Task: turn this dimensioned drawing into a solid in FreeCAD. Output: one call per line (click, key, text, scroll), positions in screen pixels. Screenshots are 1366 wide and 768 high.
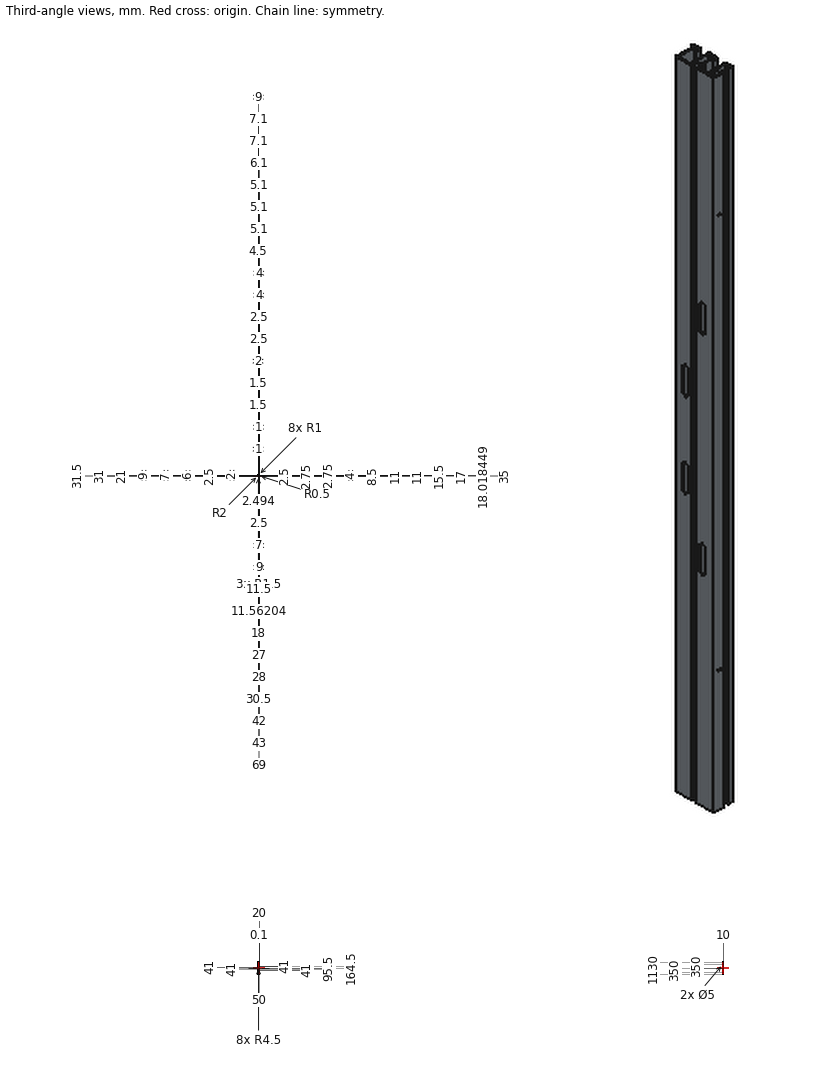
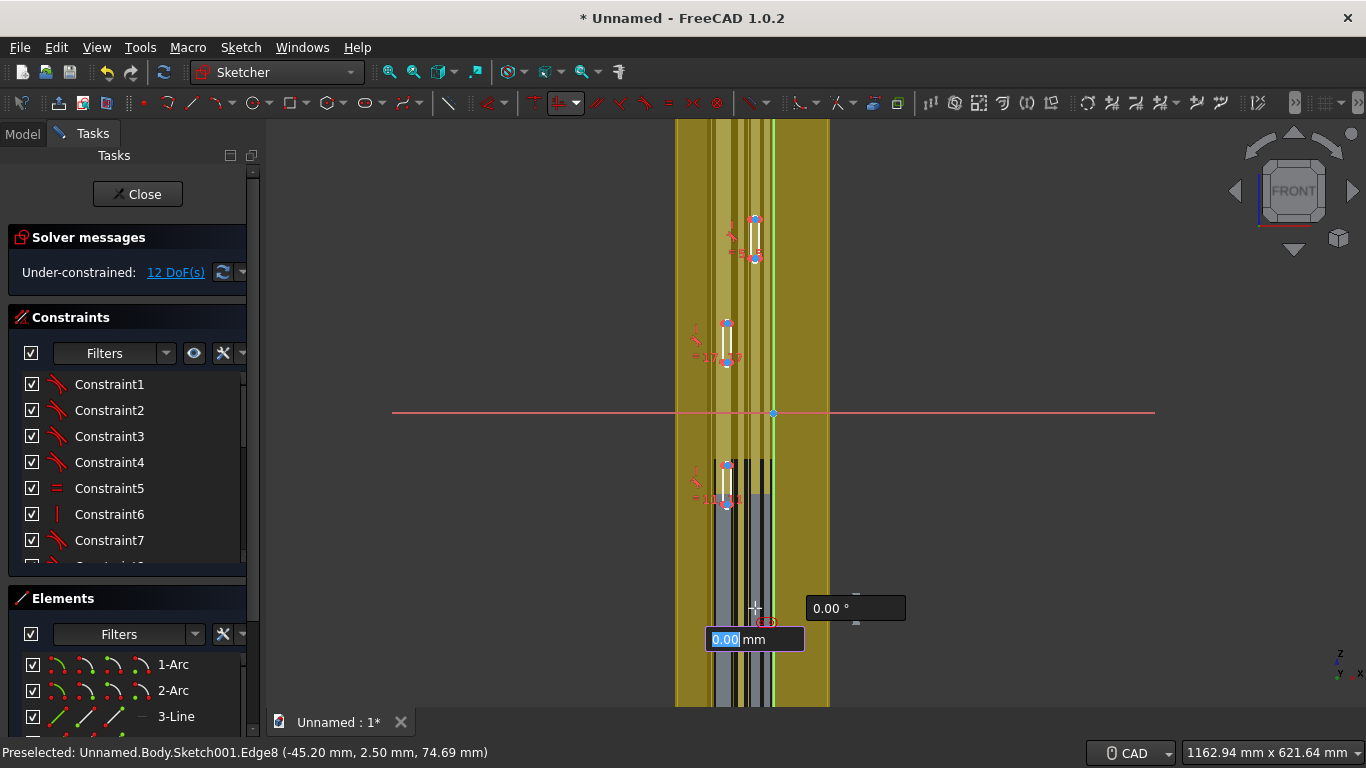
click(755, 569)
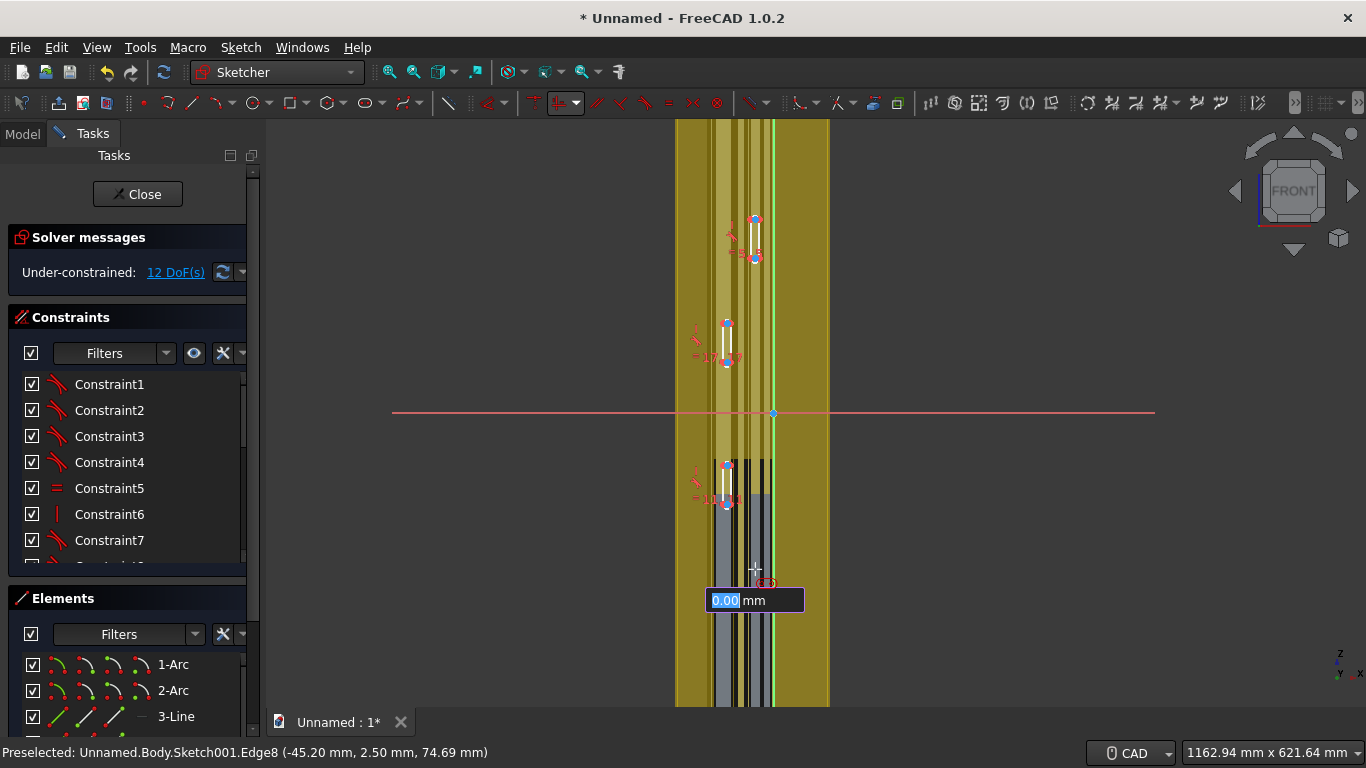
scroll(759, 588, up, 7)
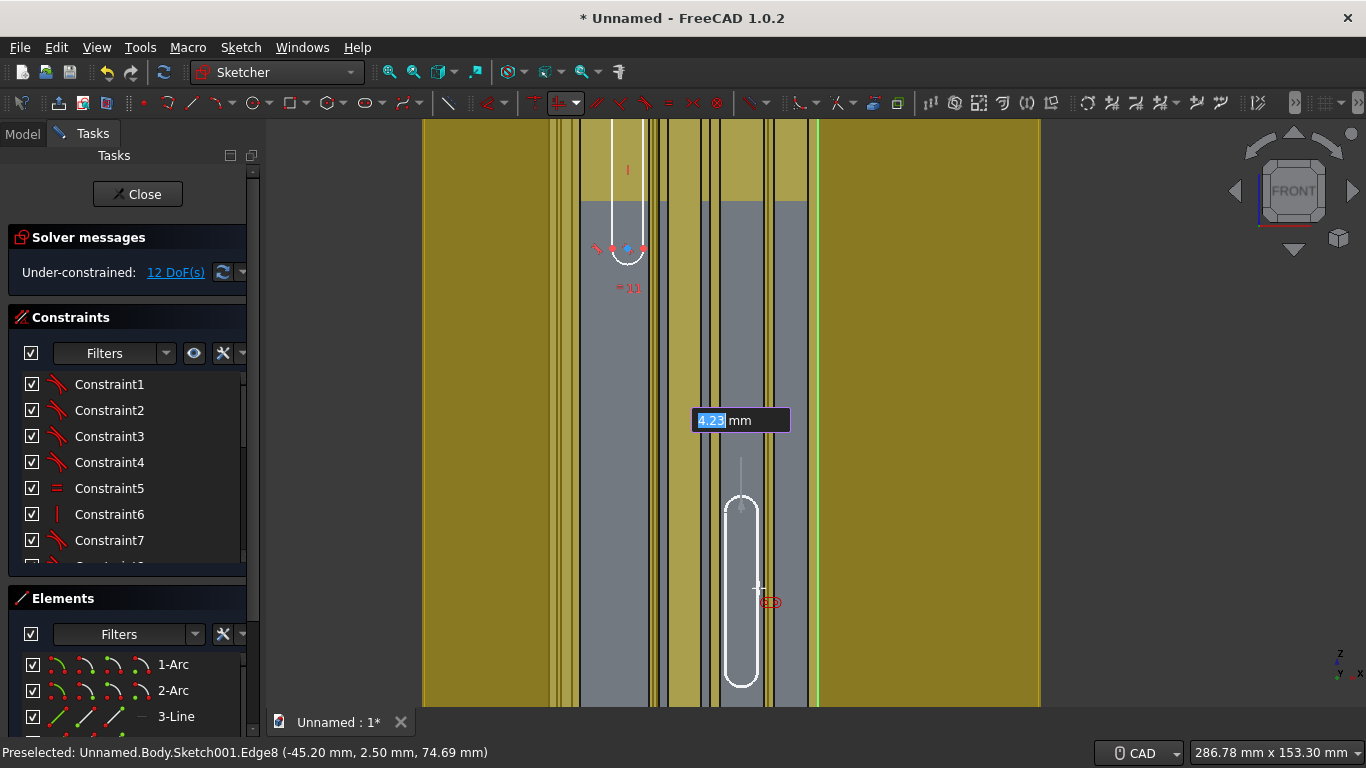
click(758, 587)
key(Escape)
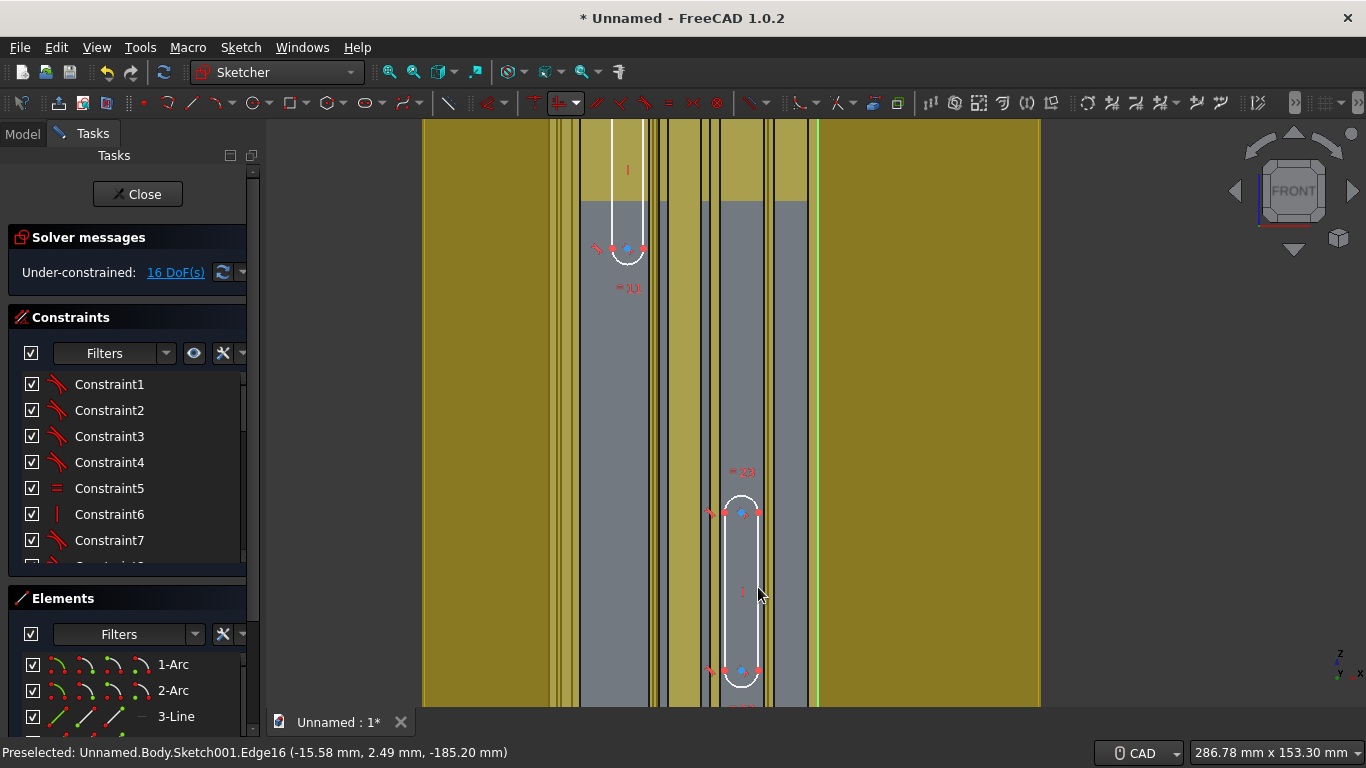
scroll(759, 588, down, 7)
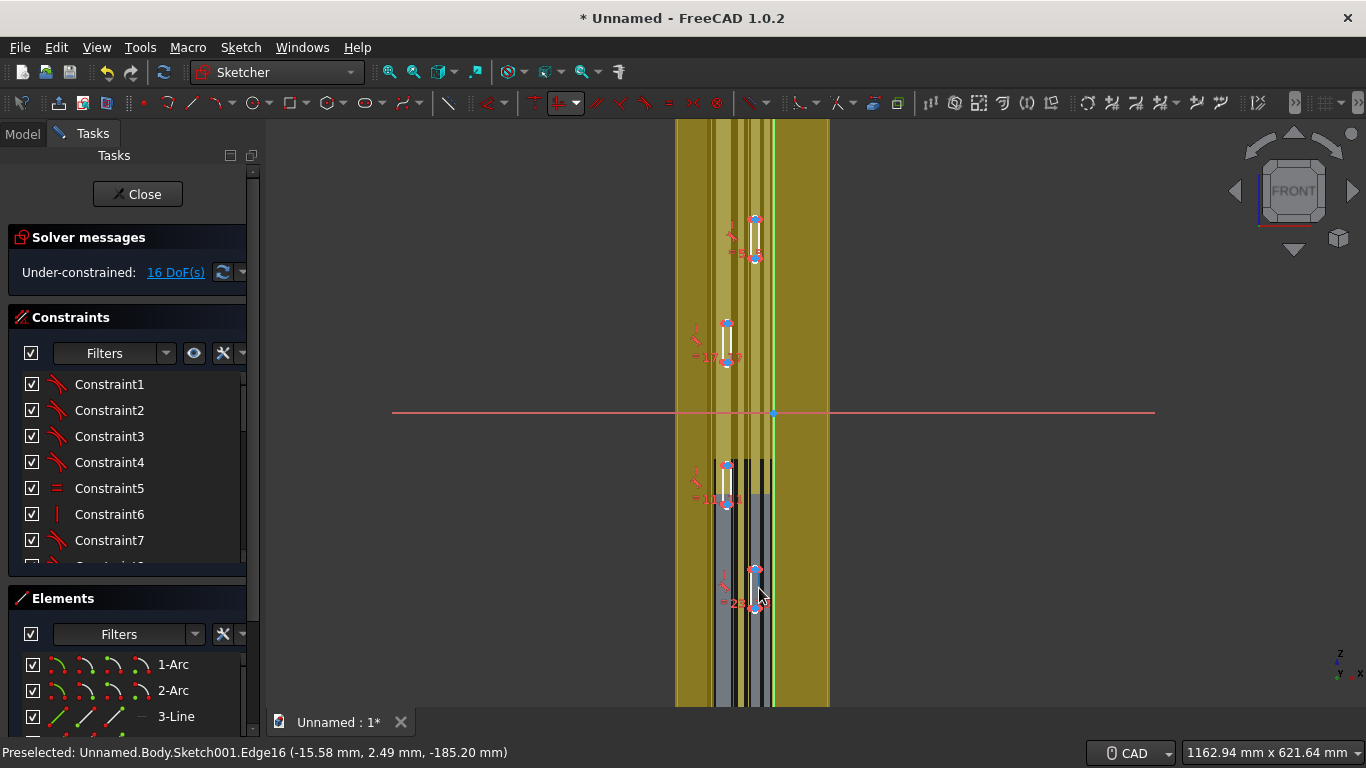
scroll(753, 262, up, 7)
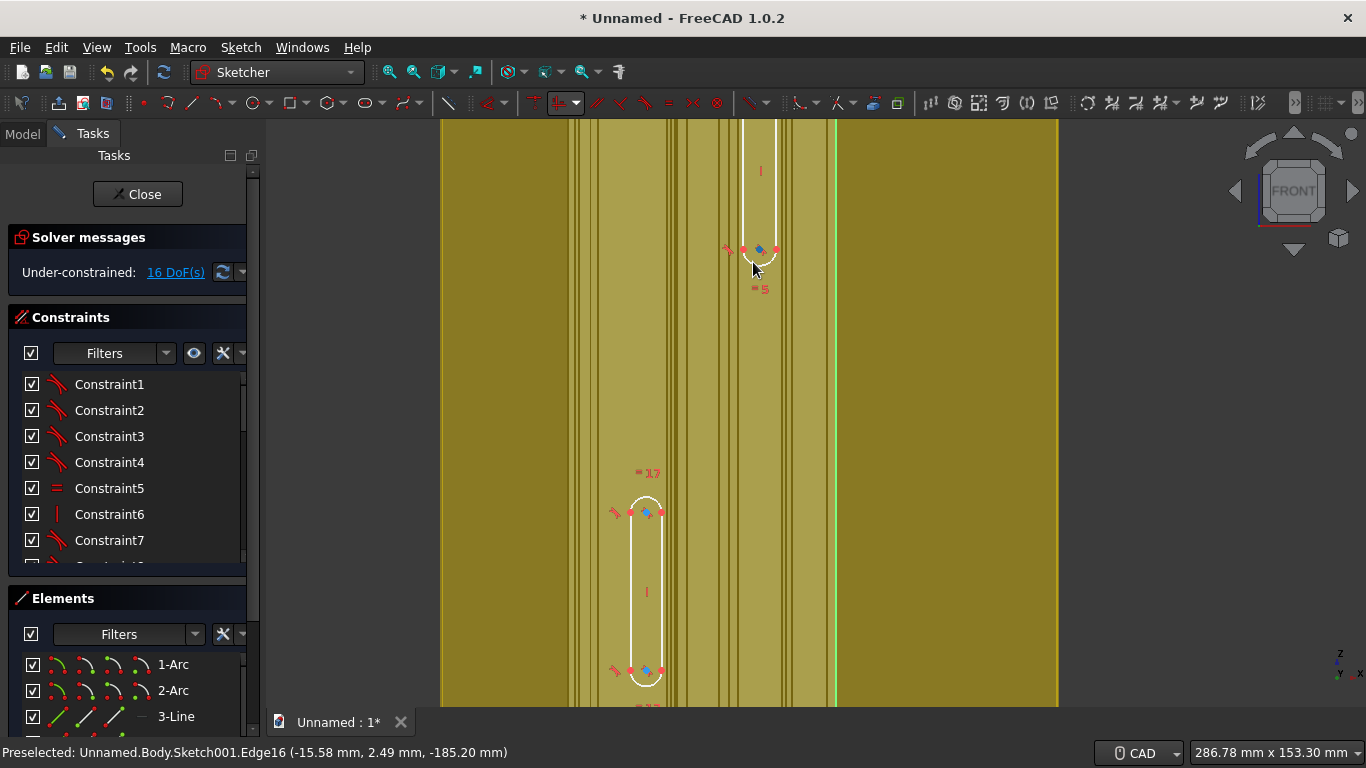
click(750, 263)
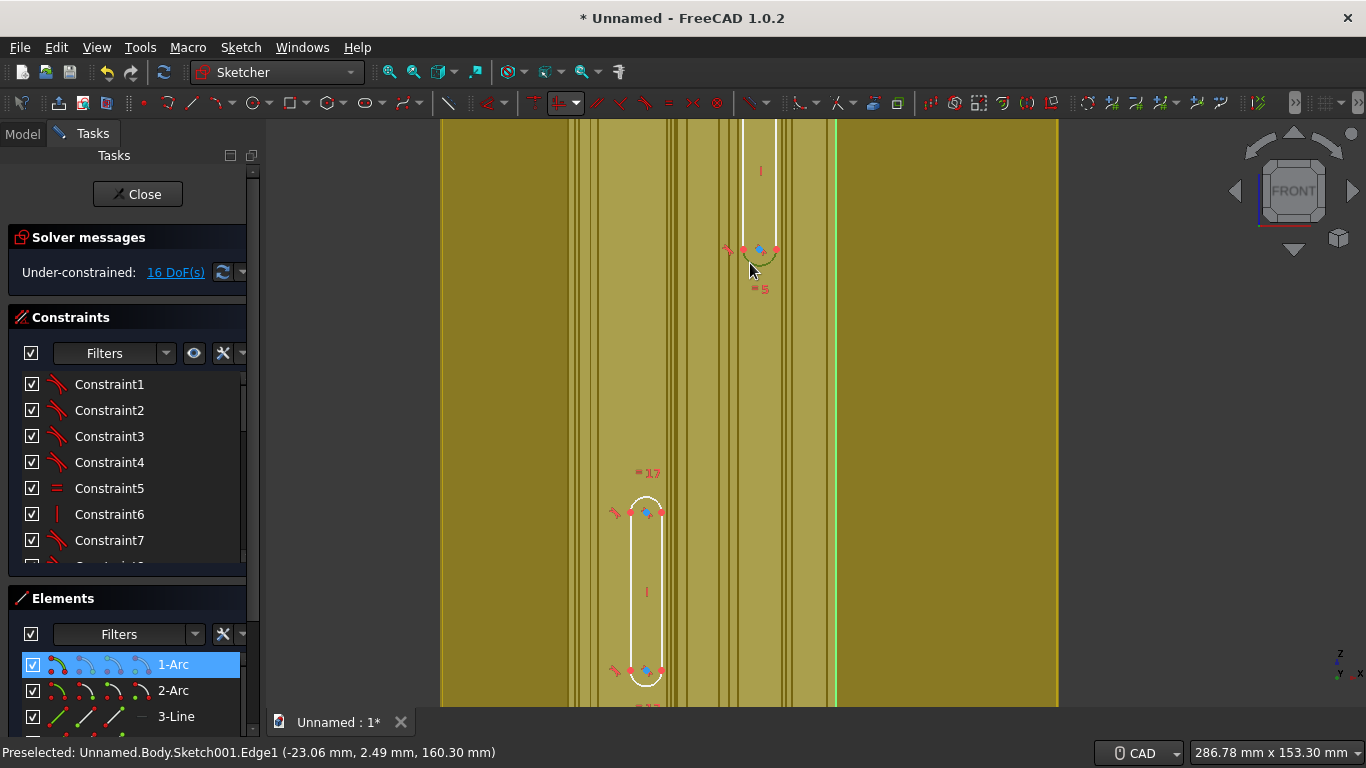
scroll(753, 262, down, 7)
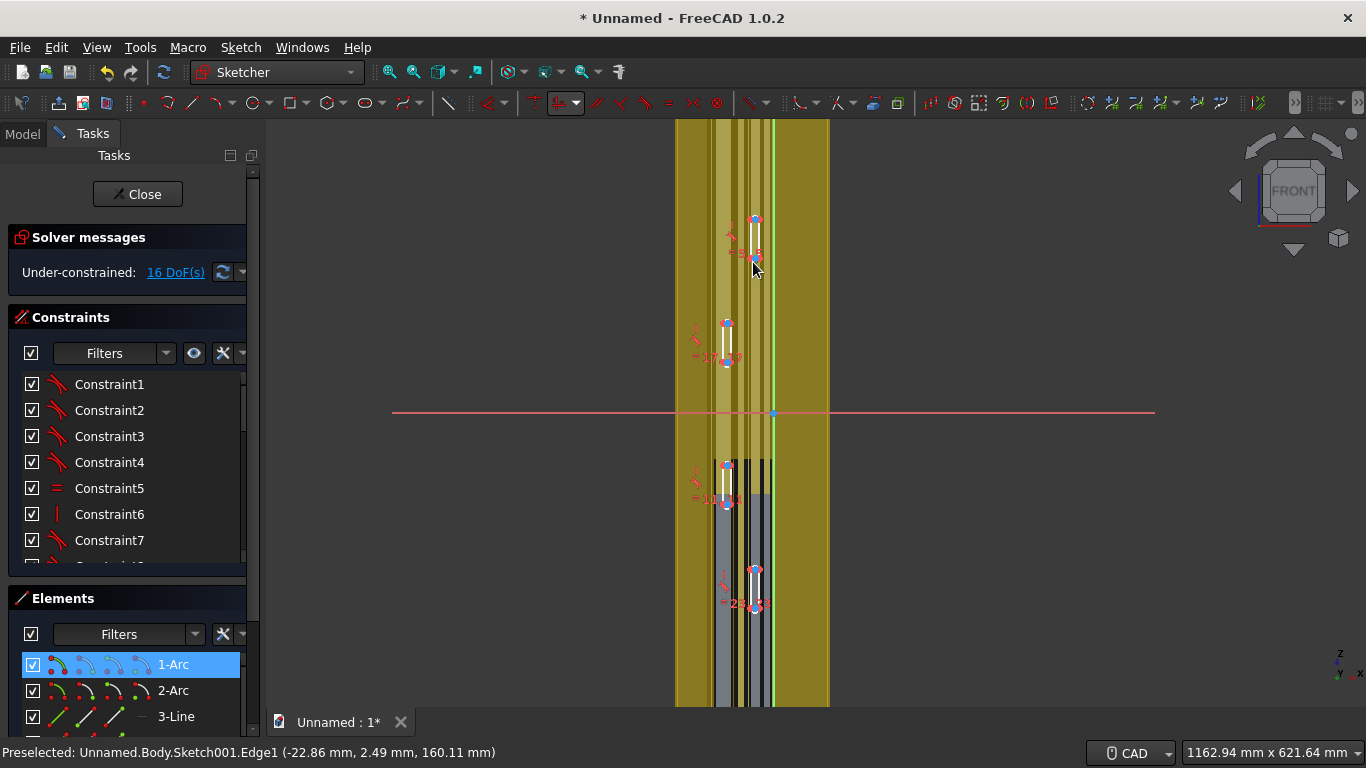
scroll(725, 508, up, 7)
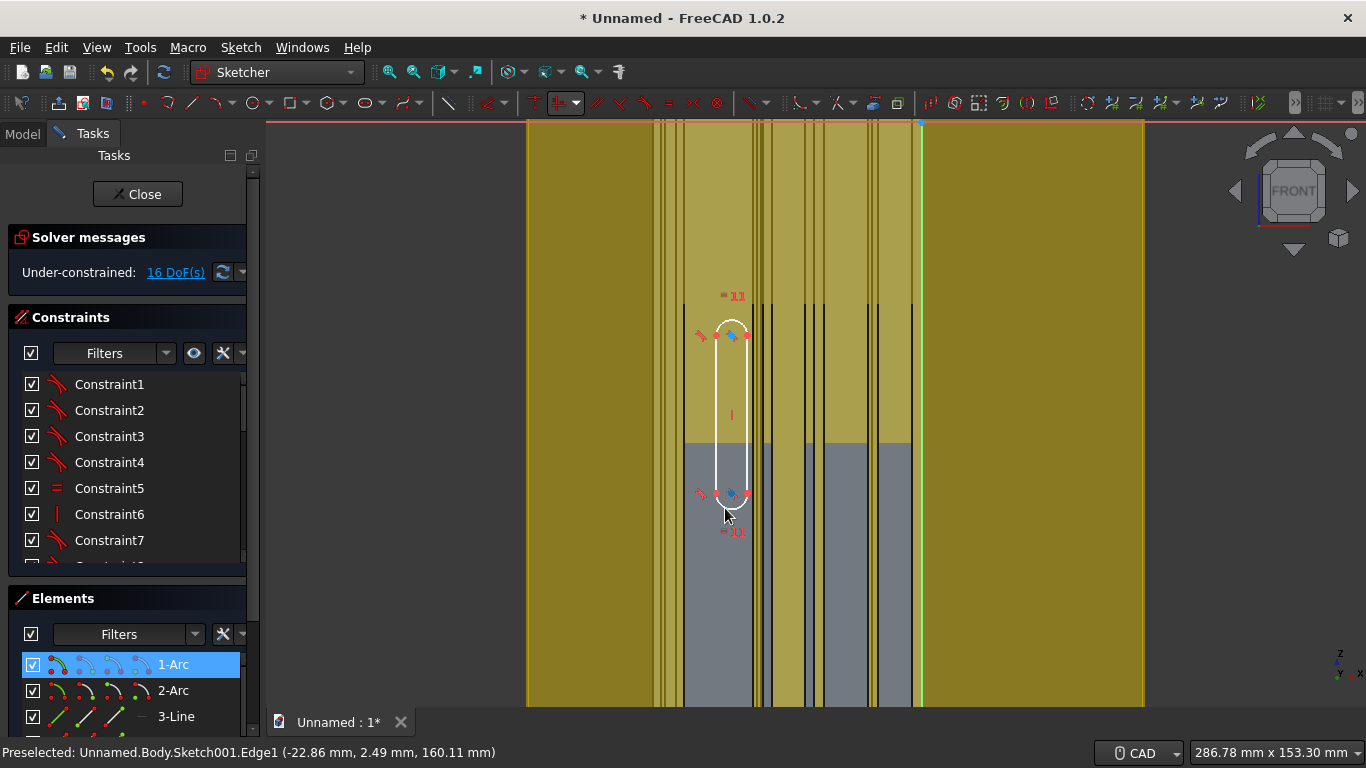
click(723, 506)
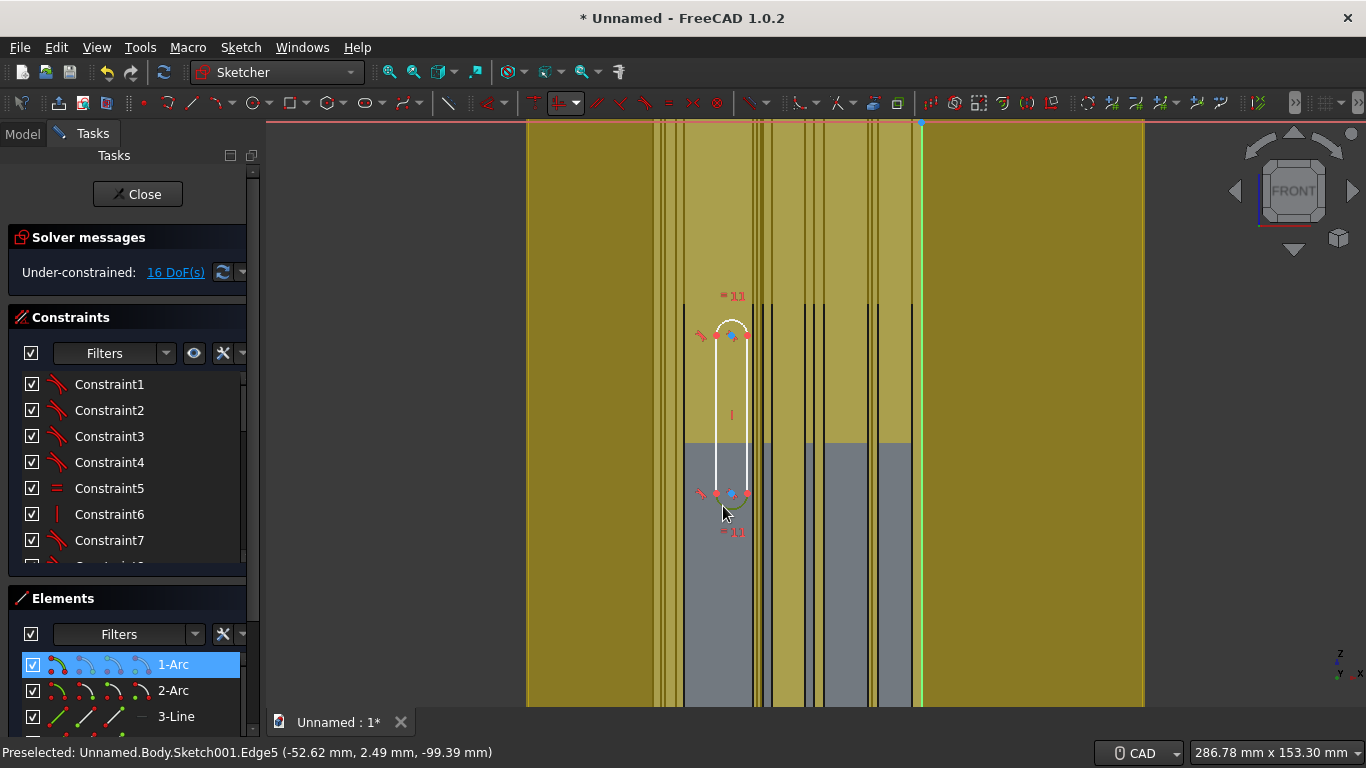
scroll(725, 508, down, 7)